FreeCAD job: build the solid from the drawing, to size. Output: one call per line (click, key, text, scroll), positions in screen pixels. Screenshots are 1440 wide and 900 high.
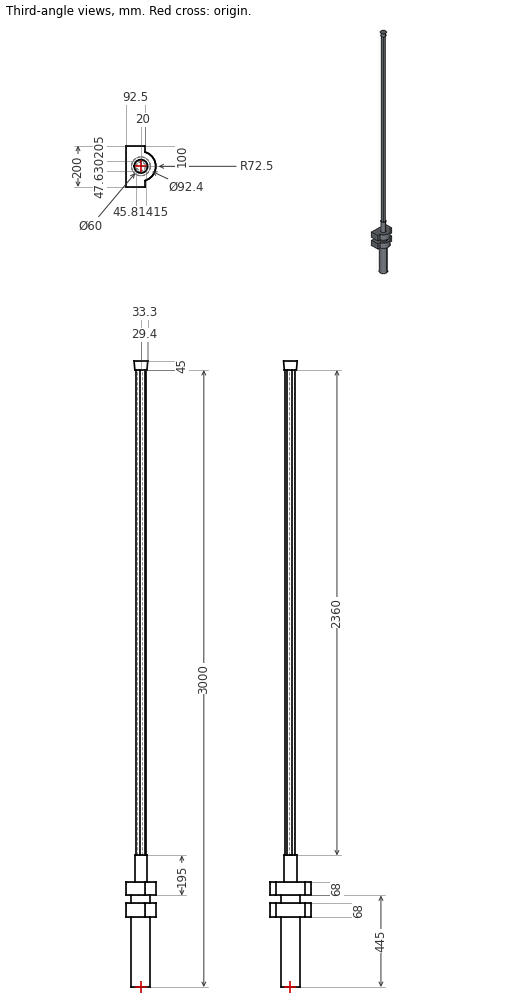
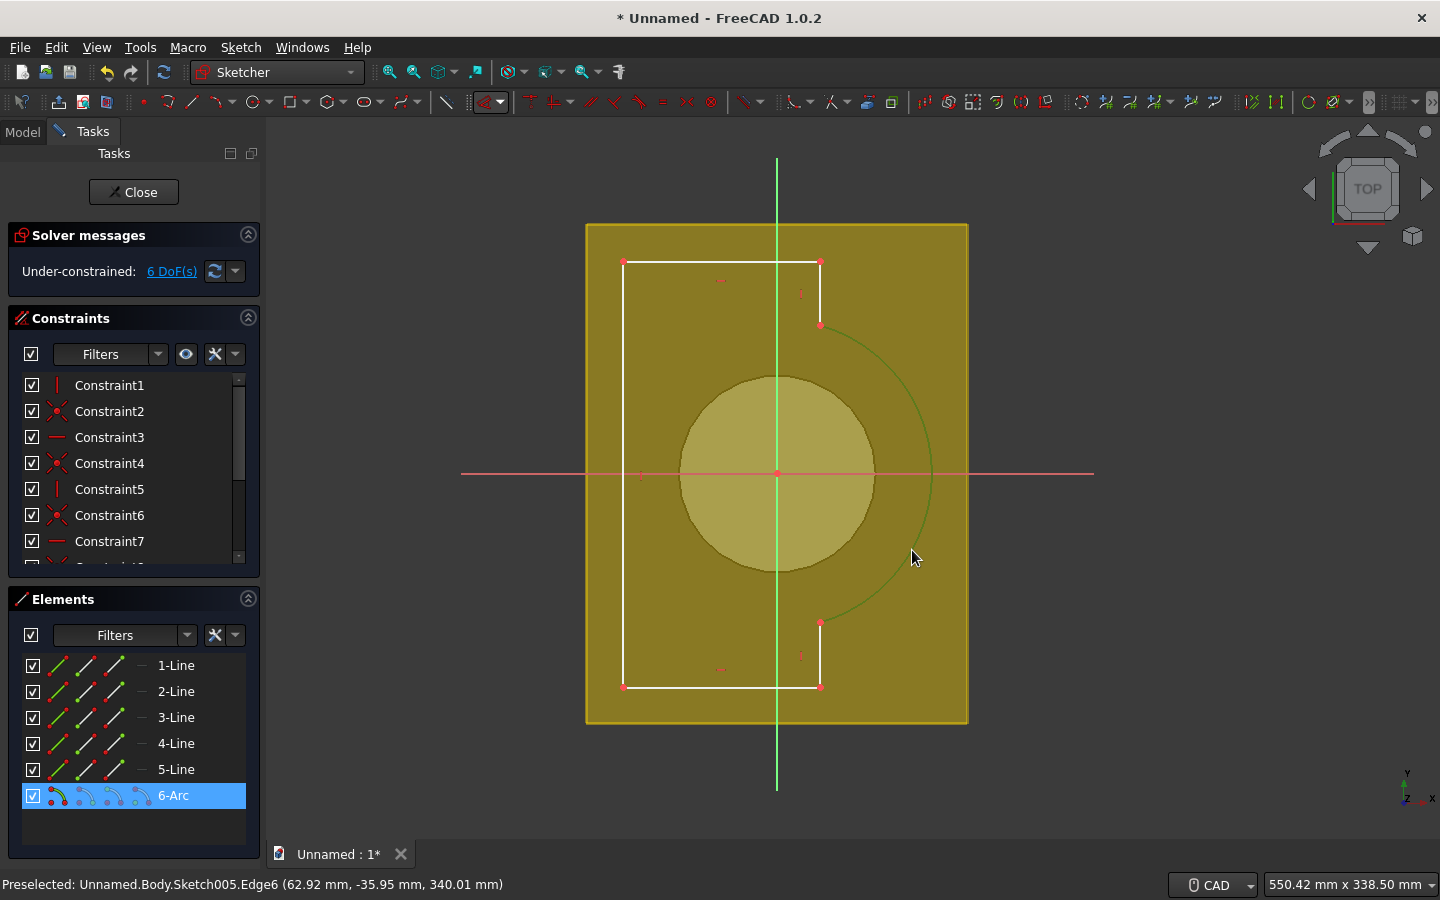
key(k)
key(r)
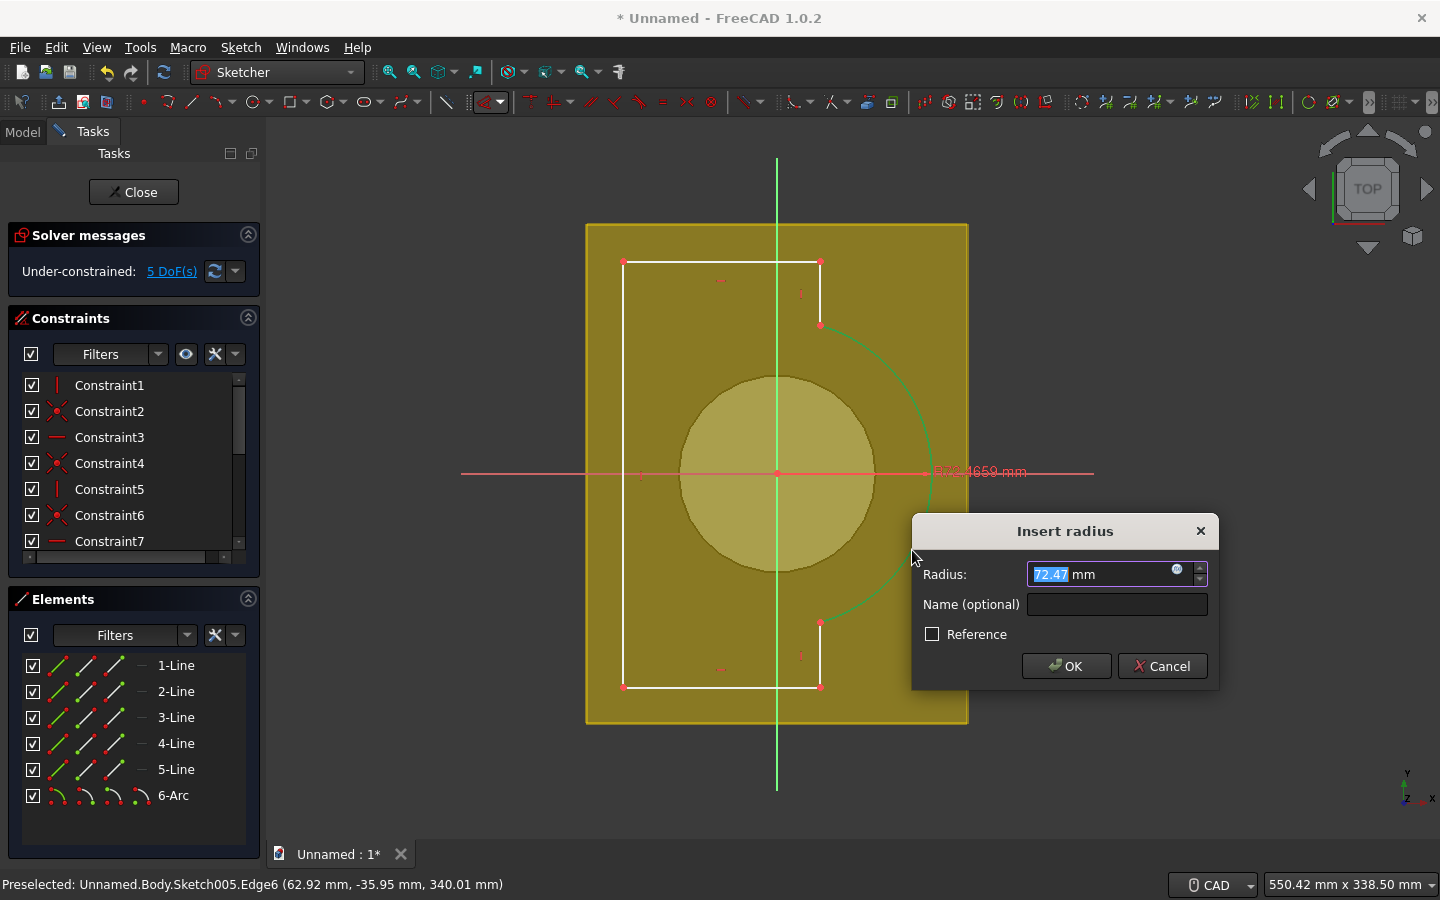
text(72.5)
key(Return)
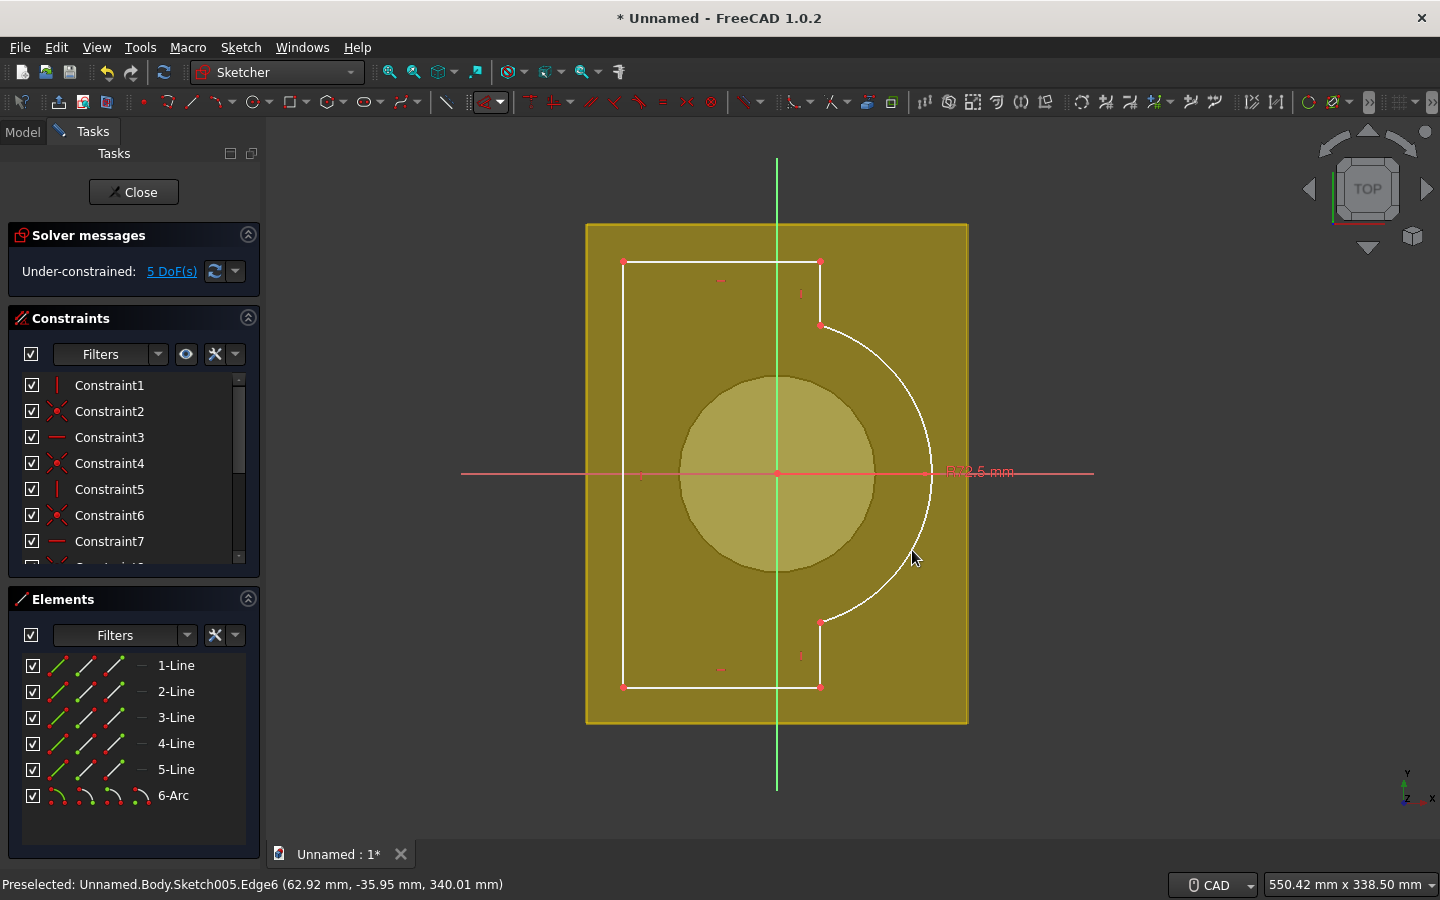
click(623, 390)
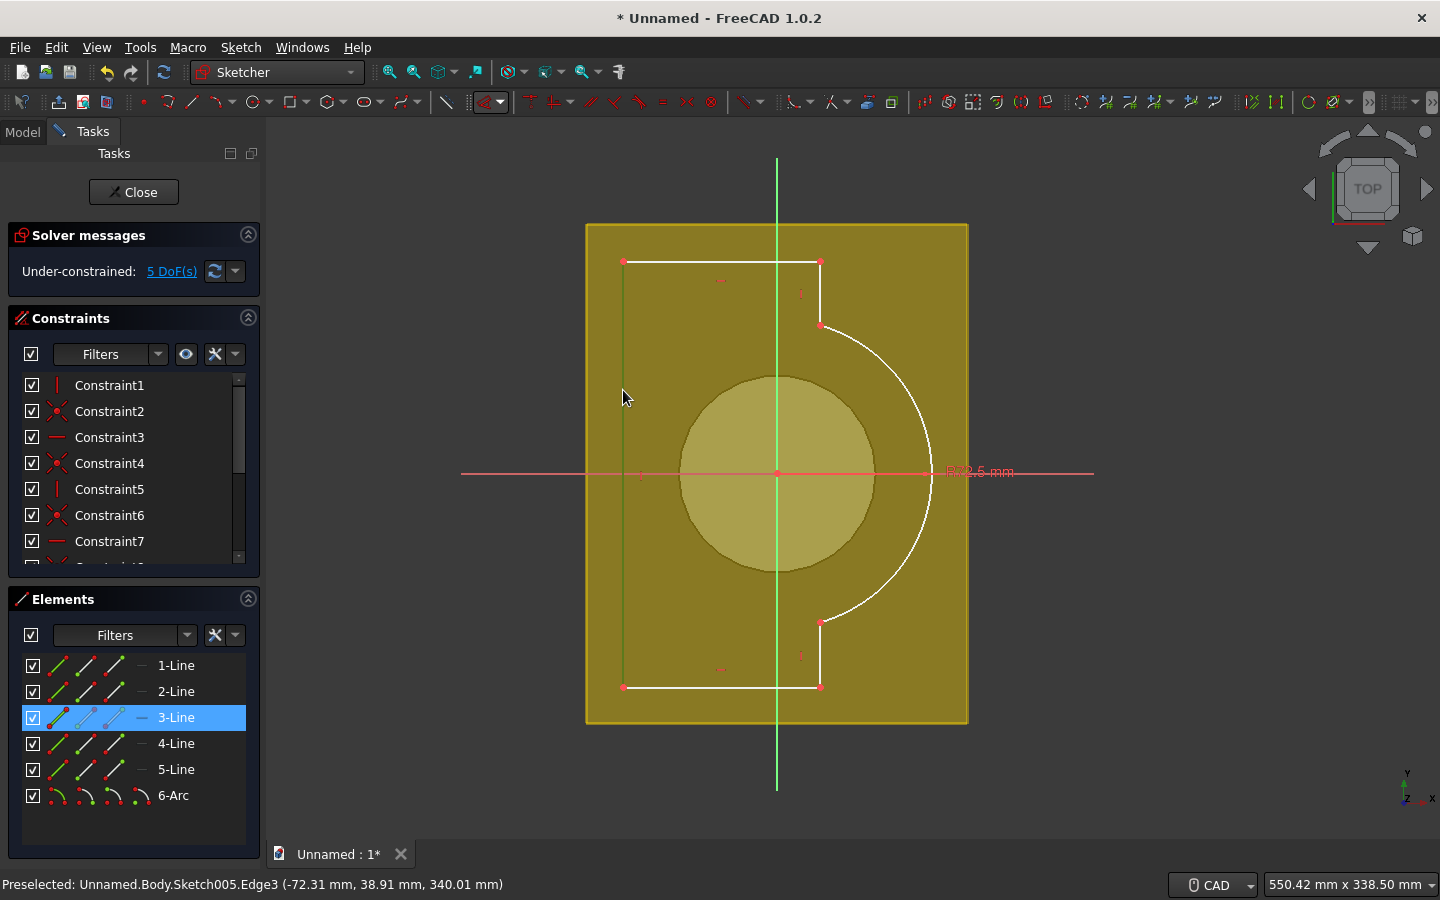
key(i)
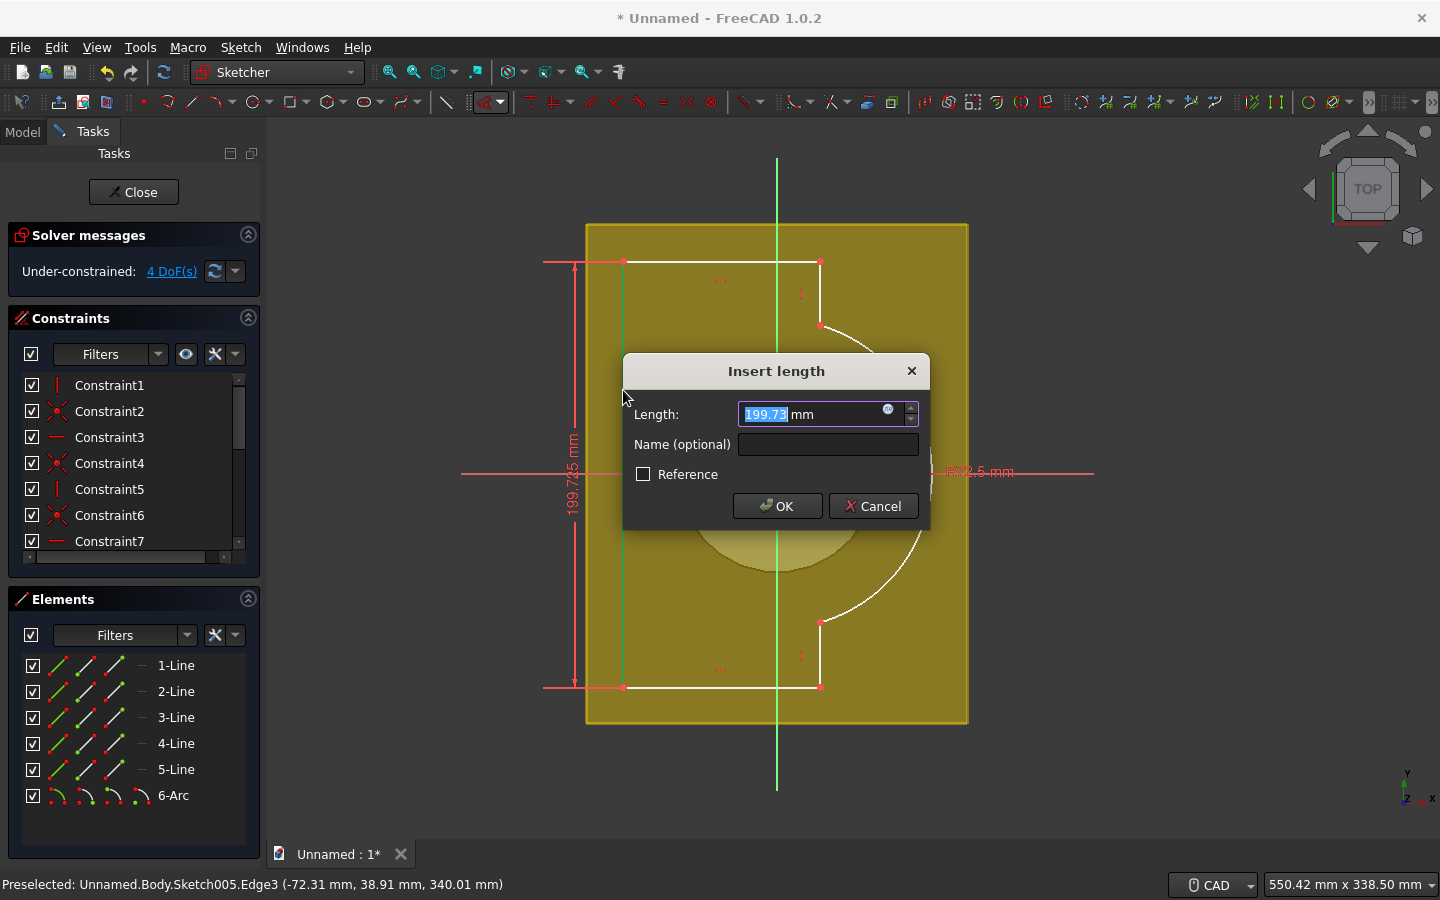
text(200)
key(Return)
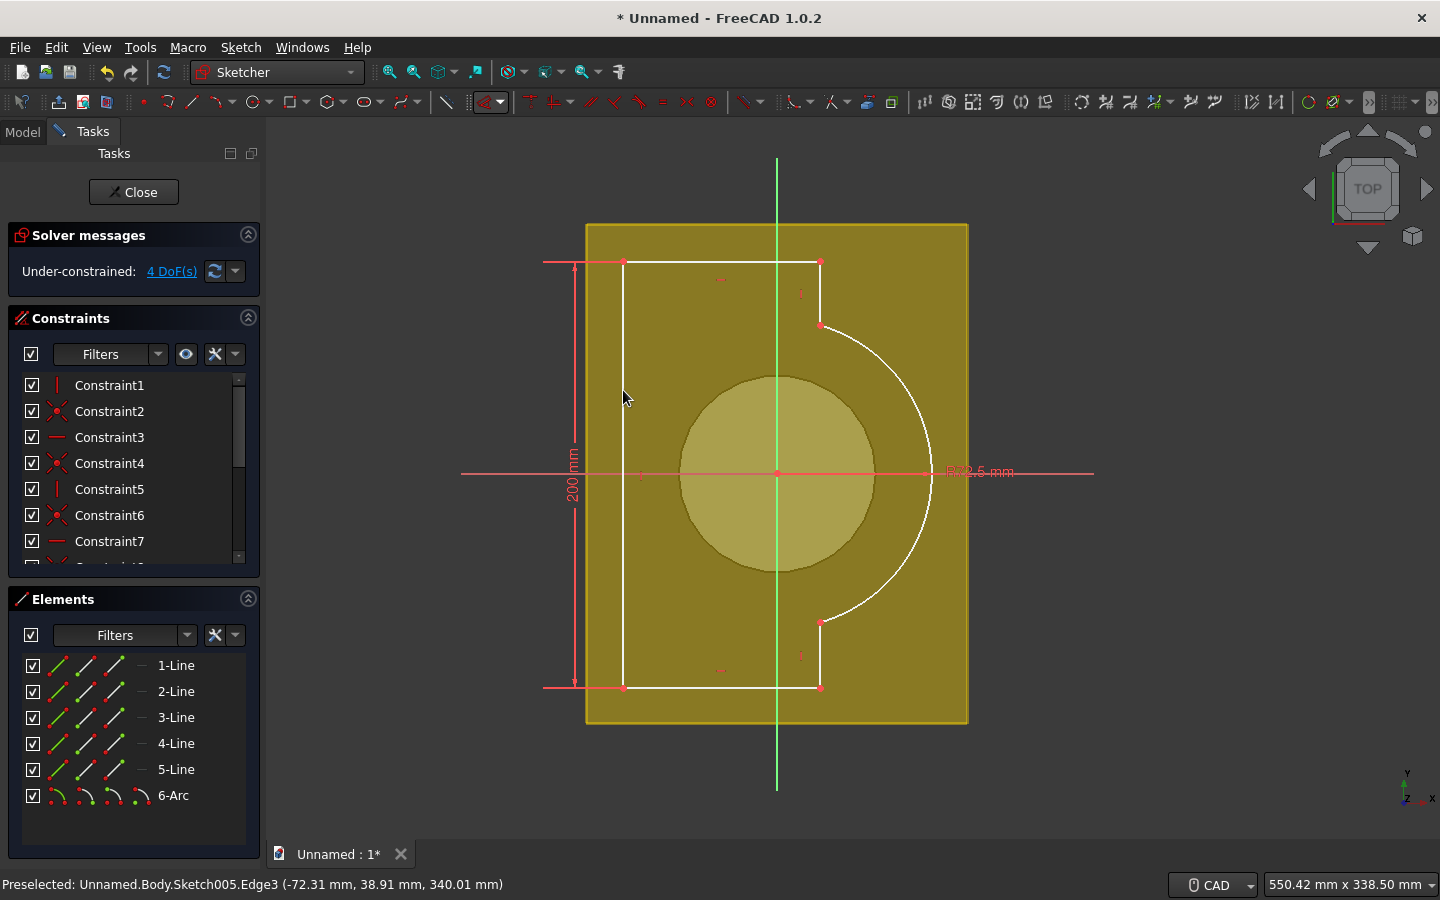
click(820, 325)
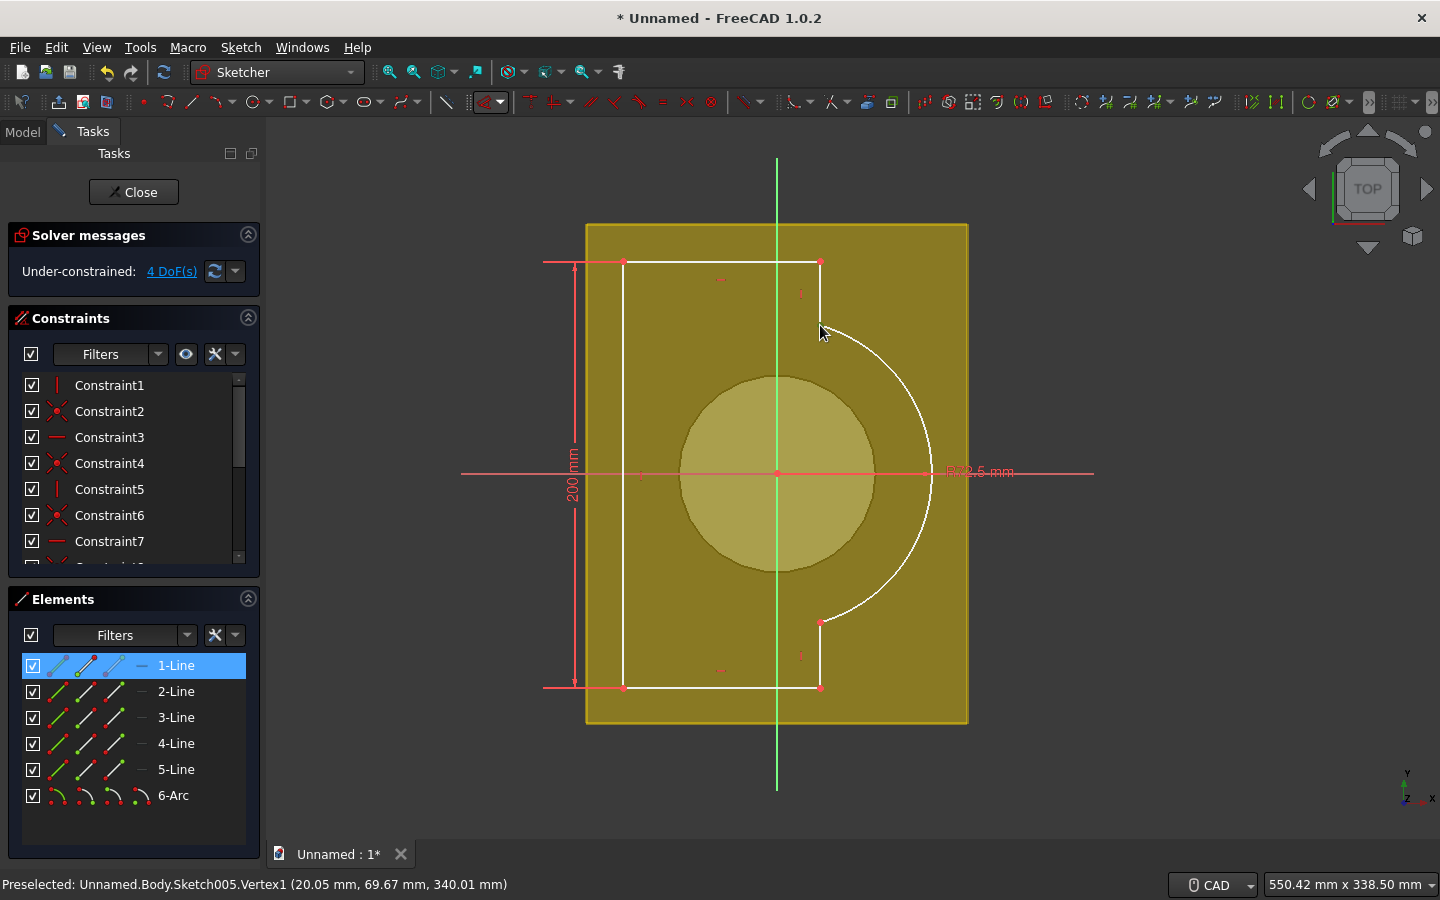
key(l)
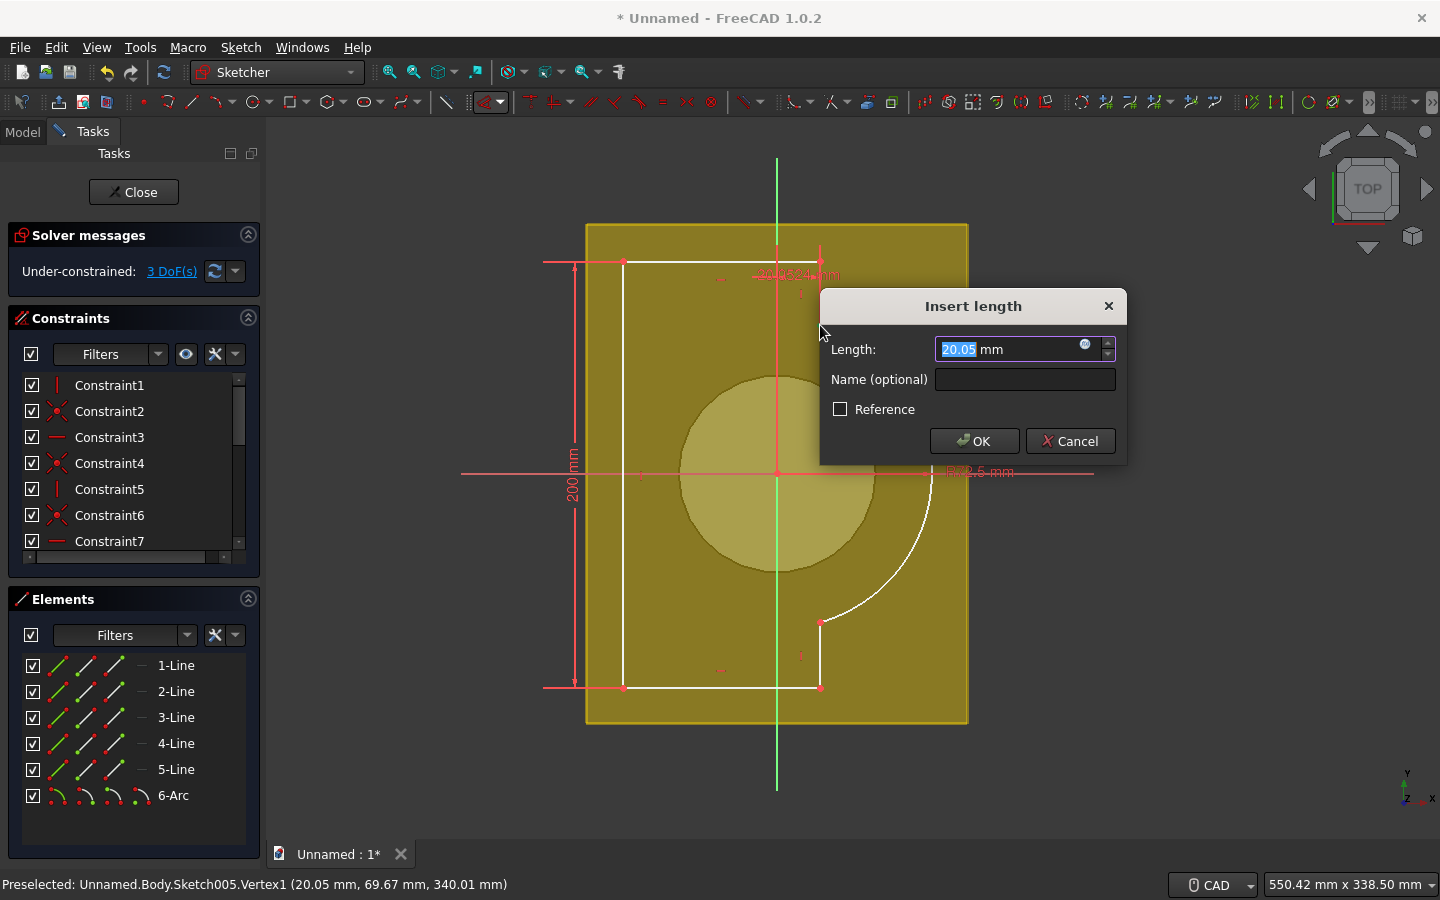
text(20)
key(Return)